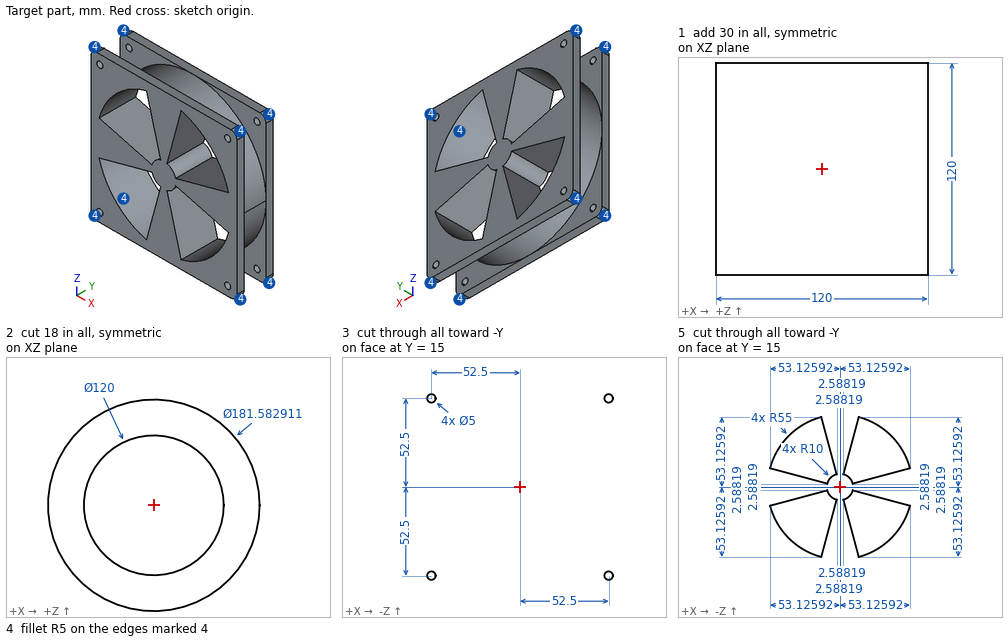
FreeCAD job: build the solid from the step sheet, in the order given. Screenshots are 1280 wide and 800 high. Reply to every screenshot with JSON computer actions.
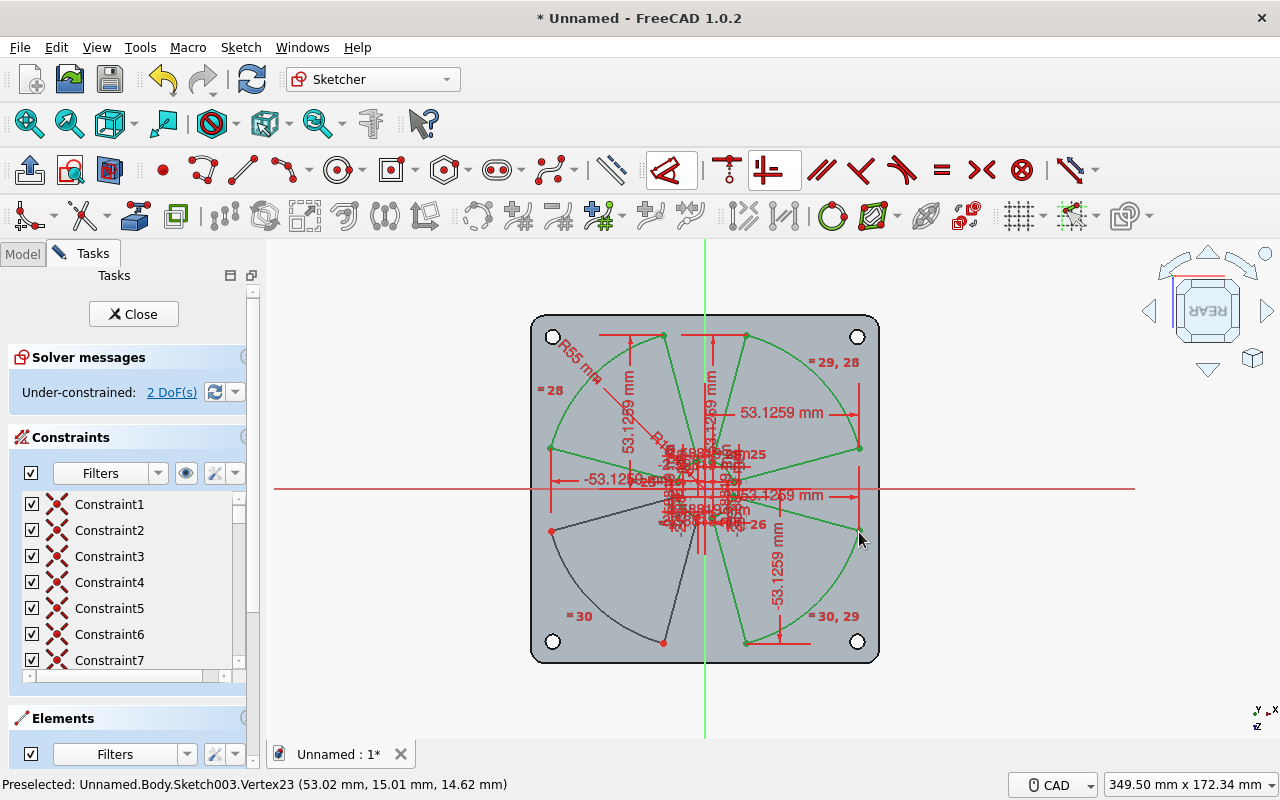
{"action": "left_click", "coordinate": [664, 644]}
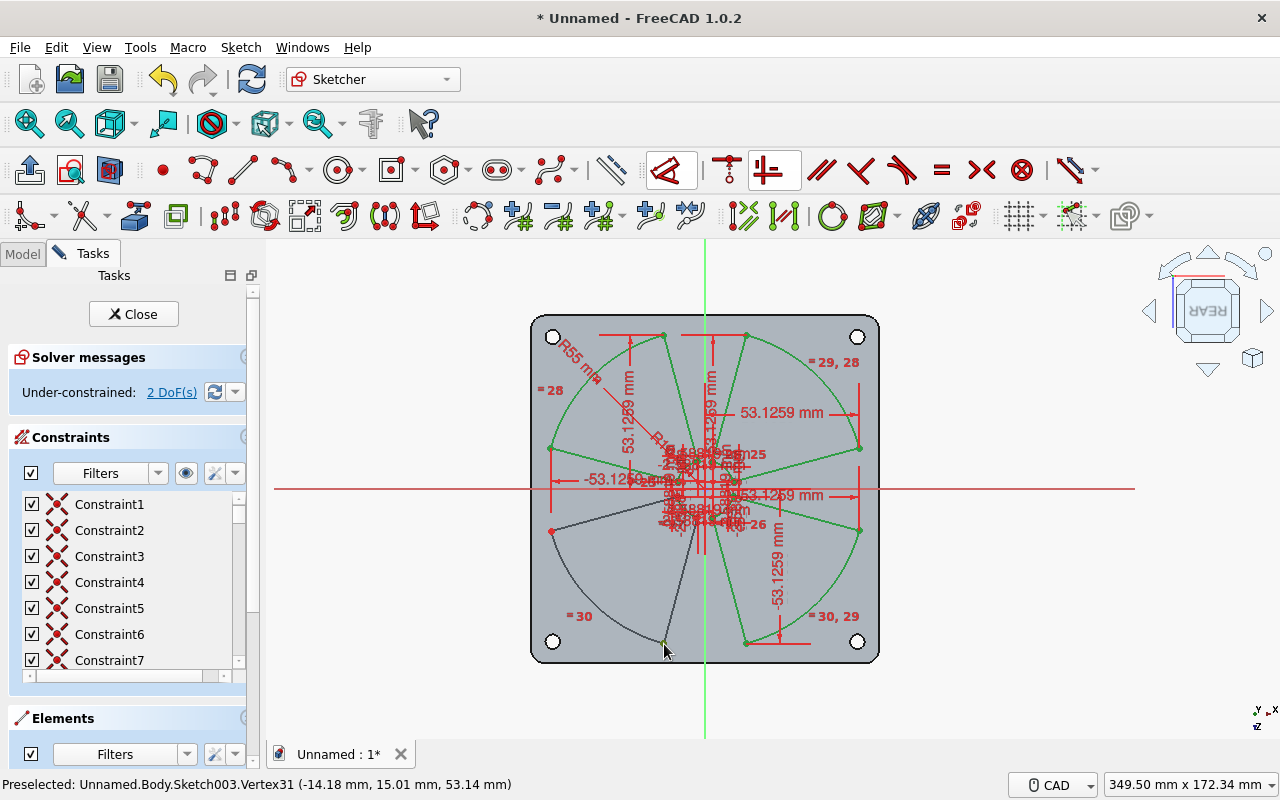
{"action": "left_click", "coordinate": [692, 170]}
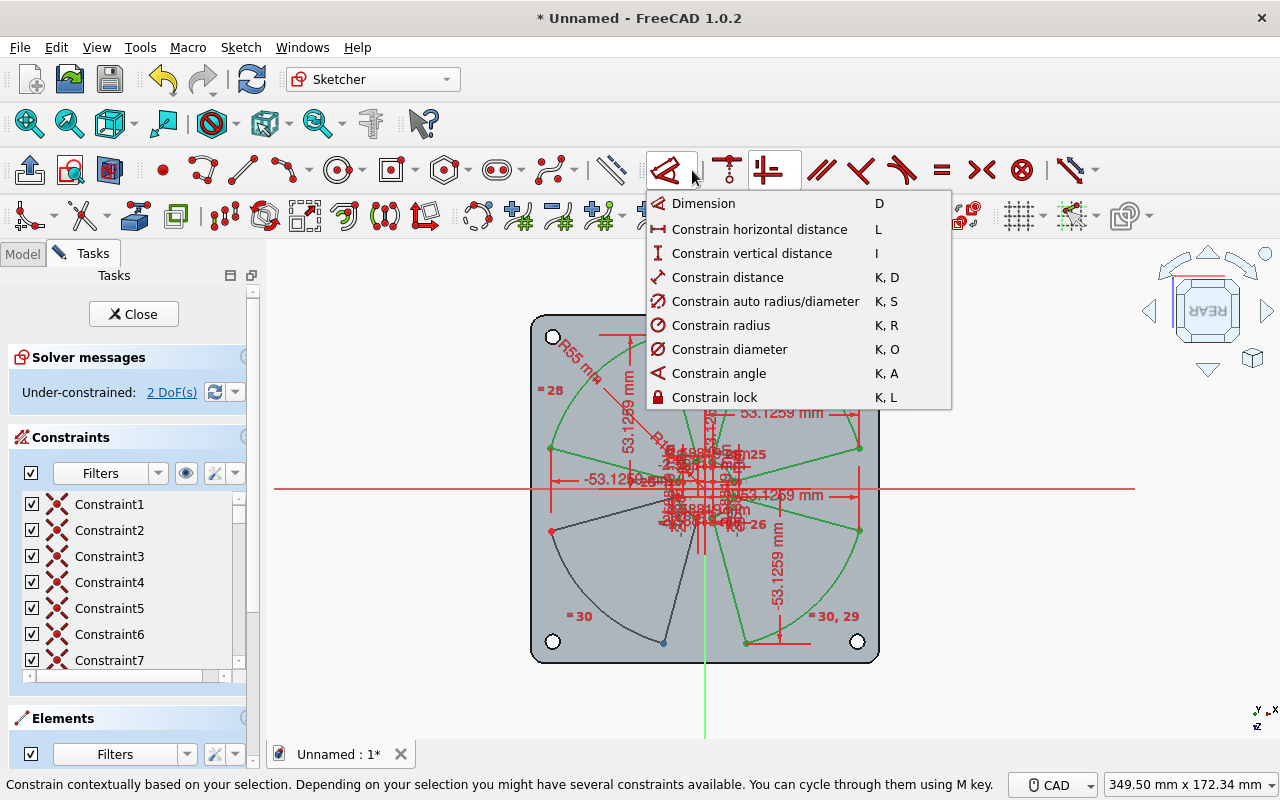
{"action": "left_click", "coordinate": [799, 253]}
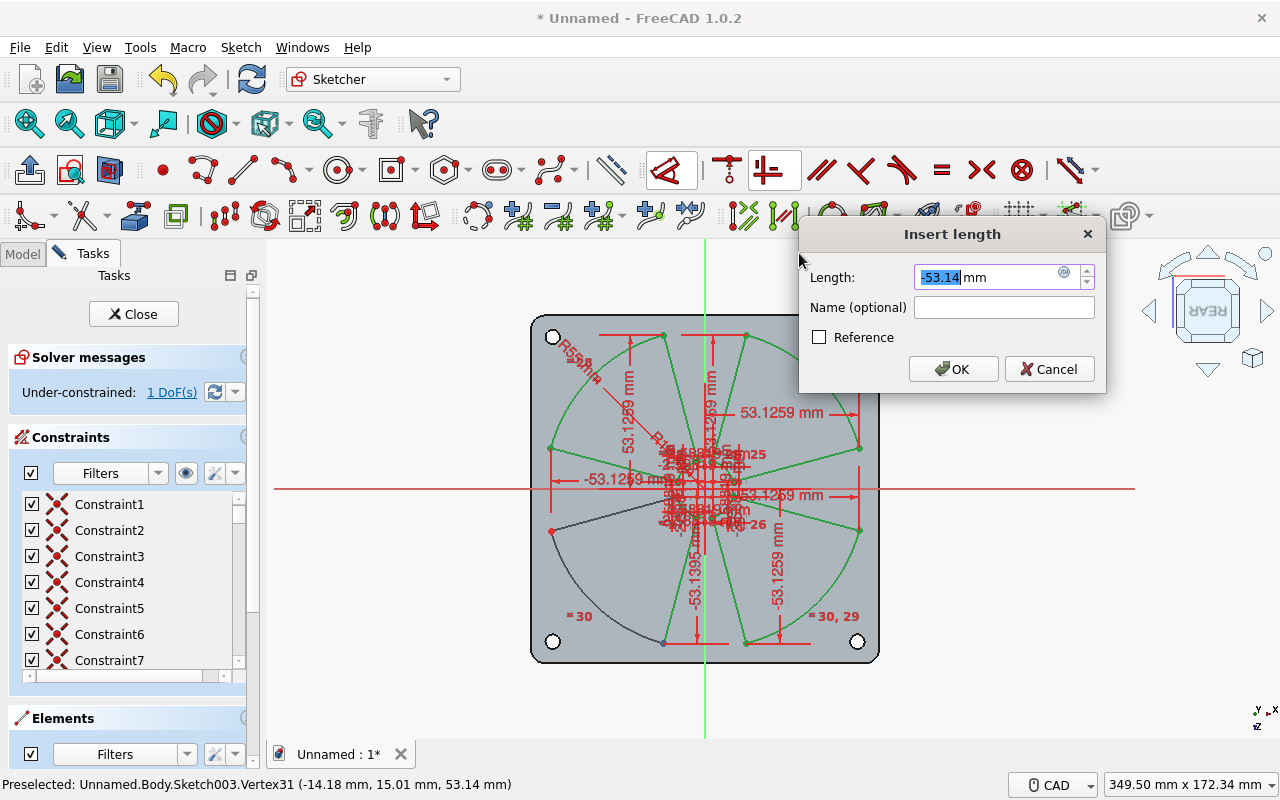
{"action": "type", "text": "-53.12592"}
{"action": "key", "text": "Return"}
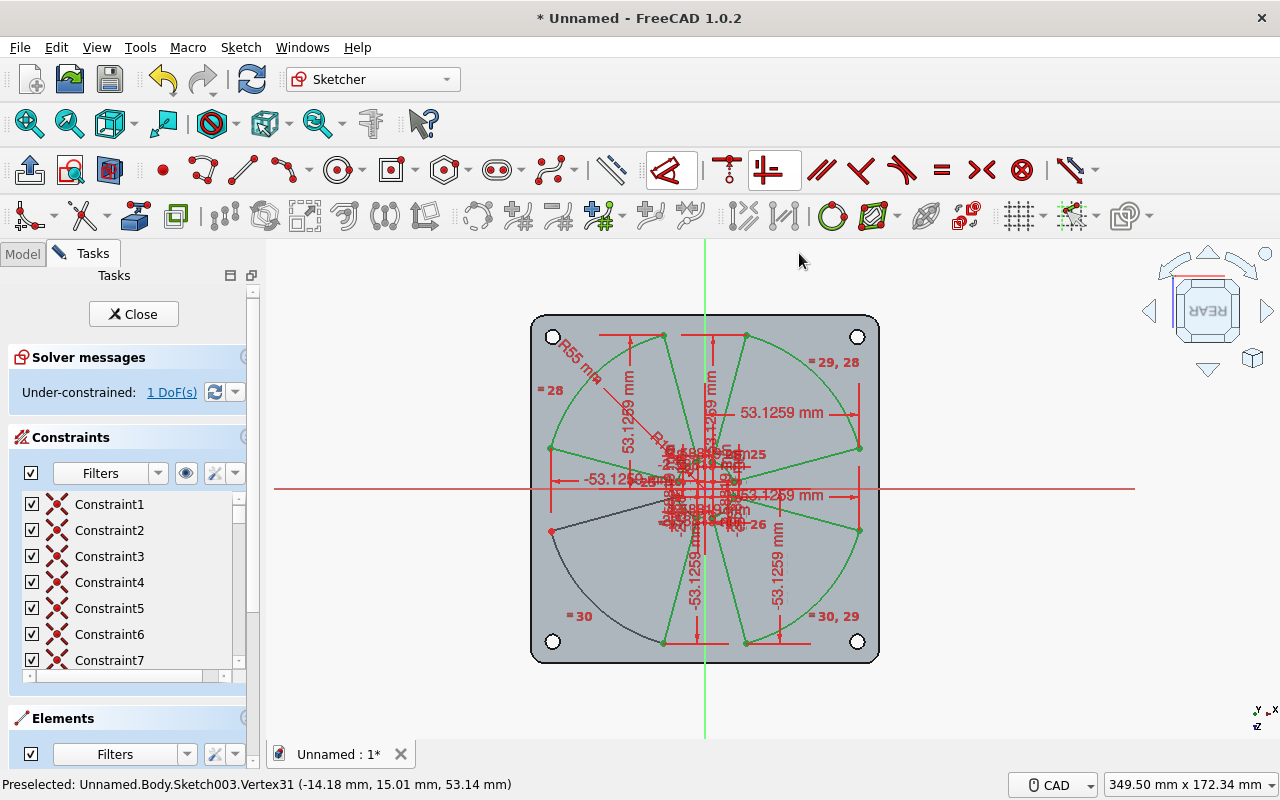
{"action": "left_click", "coordinate": [551, 531]}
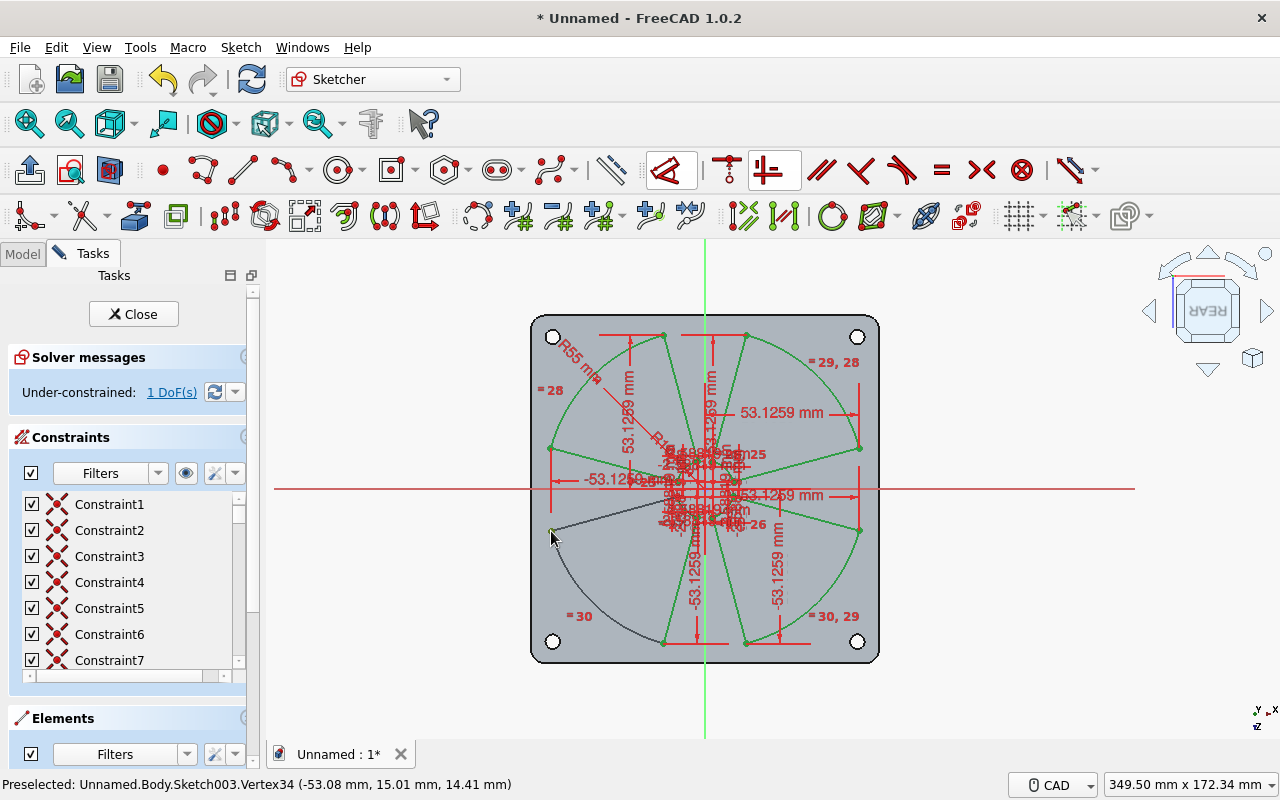
{"action": "left_click", "coordinate": [692, 170]}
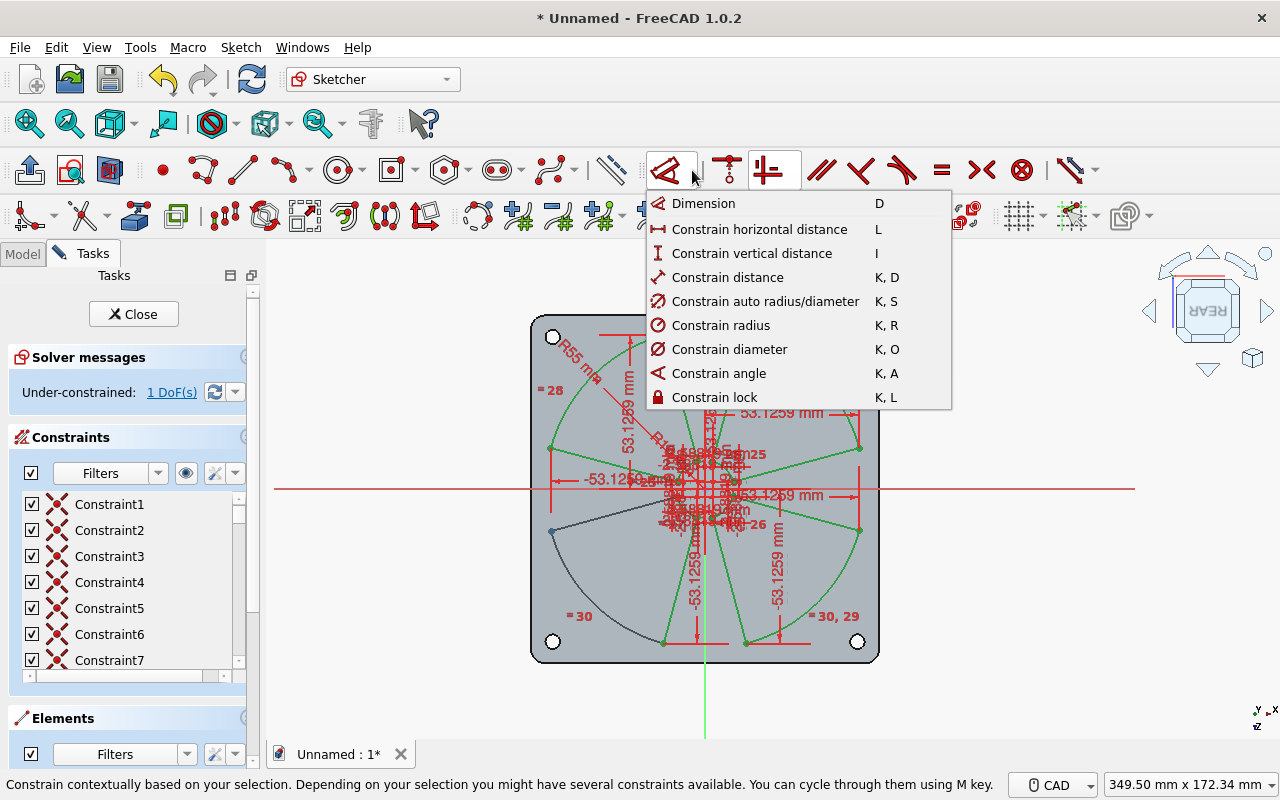
{"action": "left_click", "coordinate": [799, 229]}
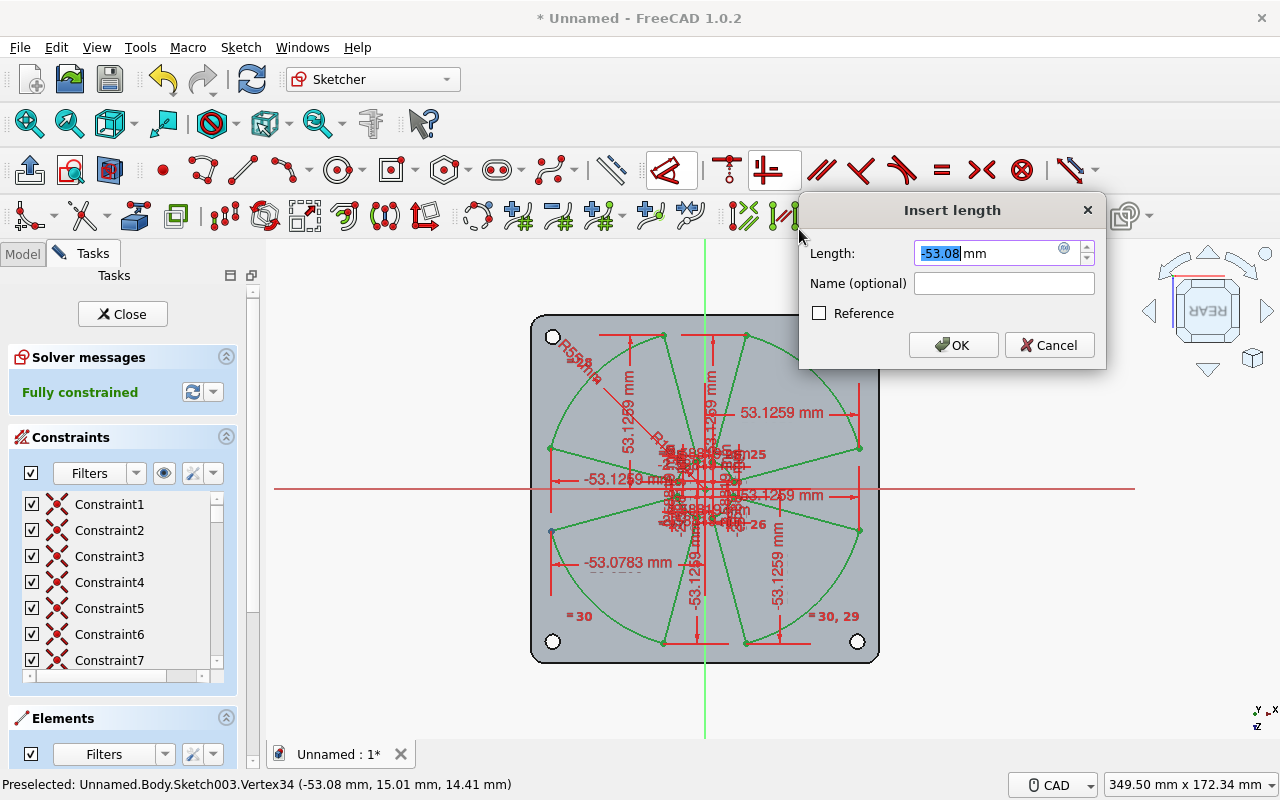
{"action": "type", "text": "-53.12592"}
{"action": "key", "text": "Return"}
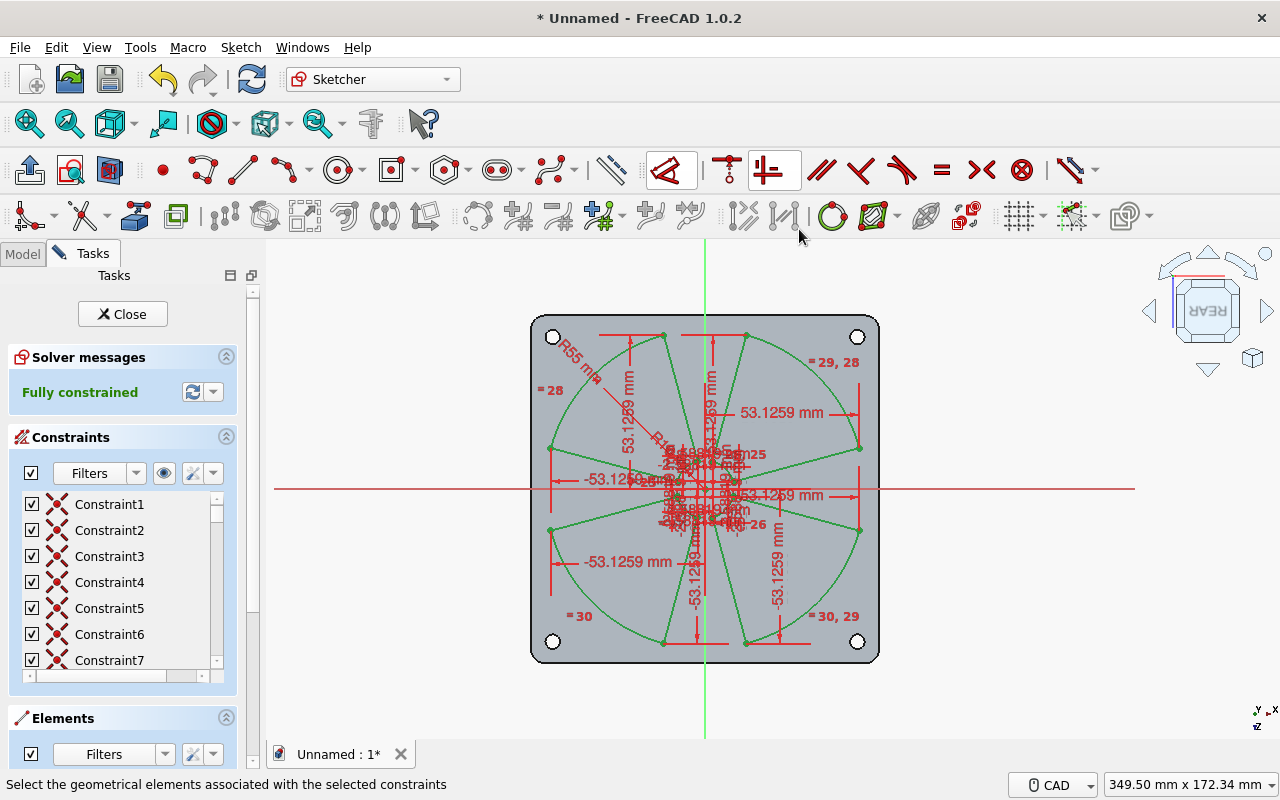
{"action": "left_click", "coordinate": [123, 314]}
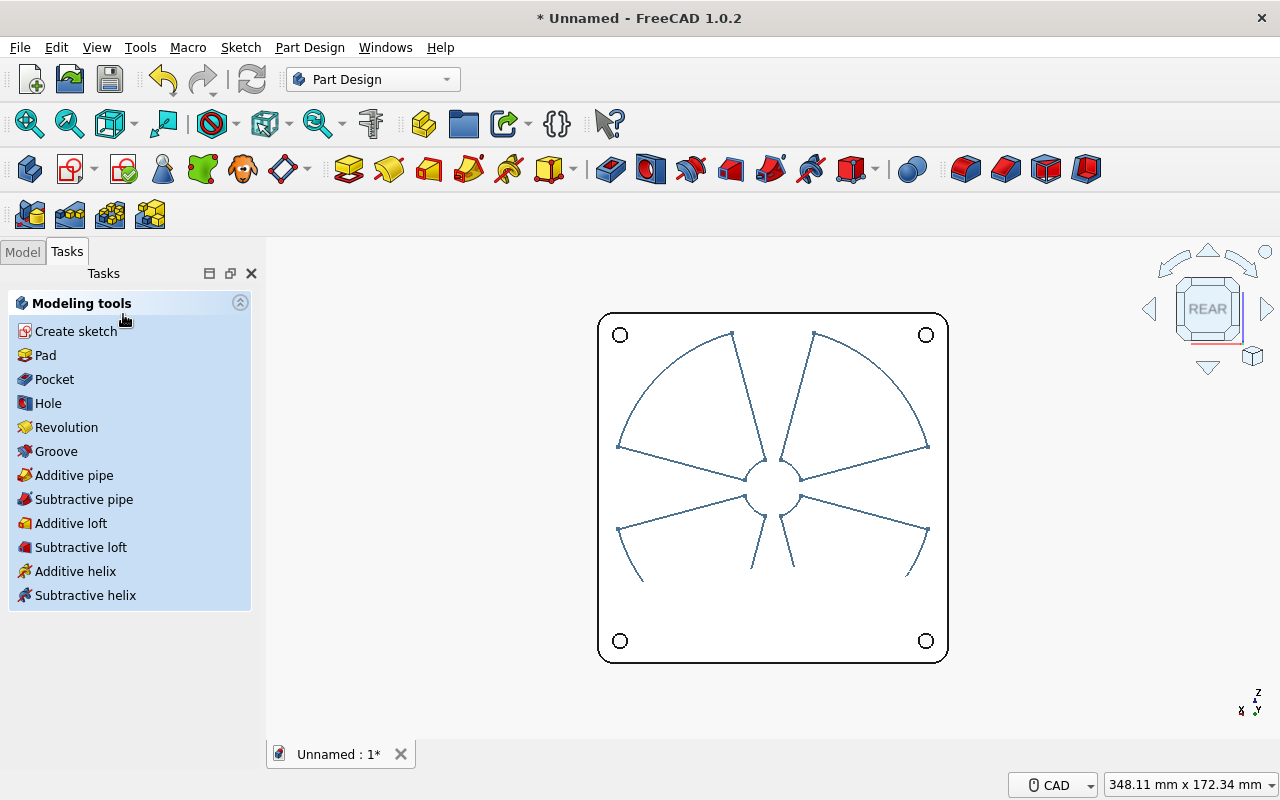
{"action": "left_click", "coordinate": [612, 170]}